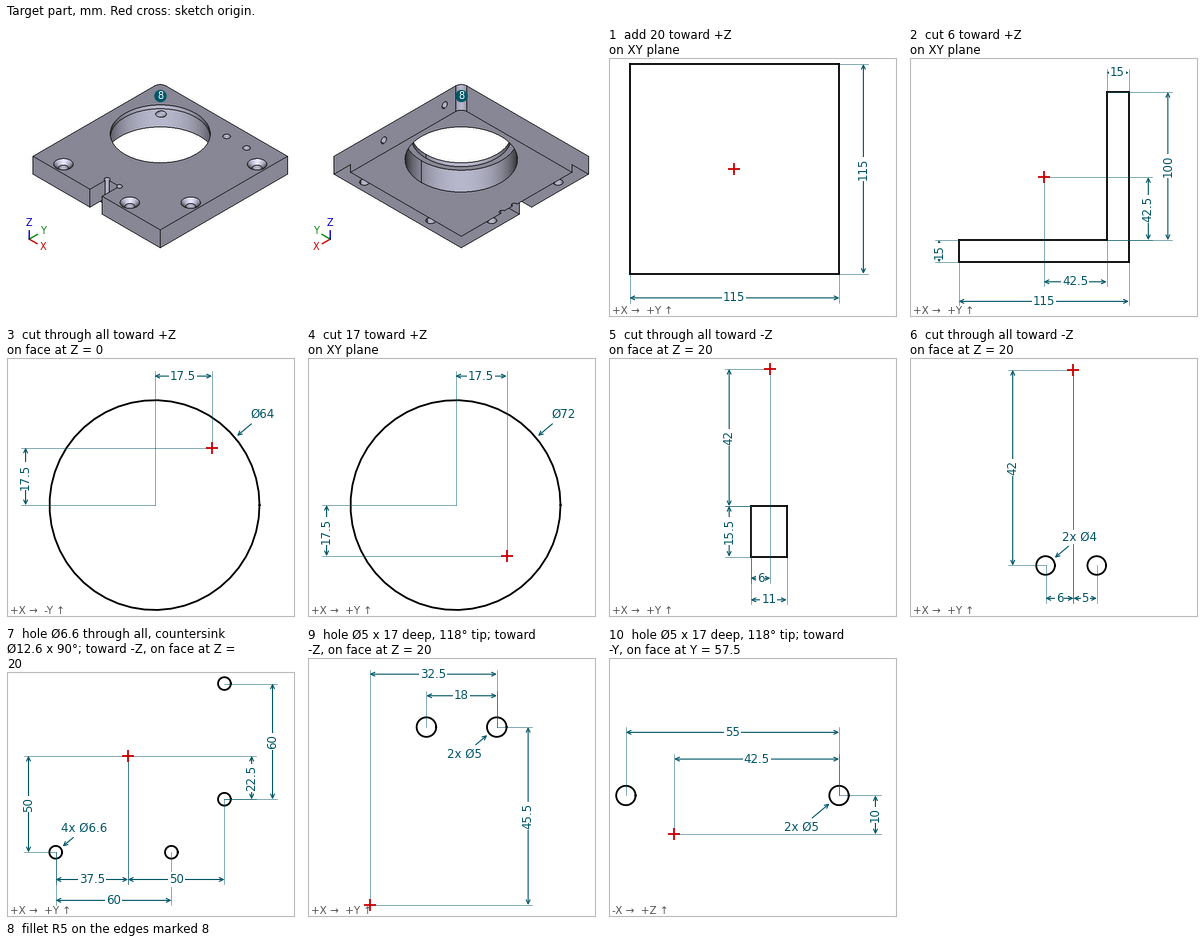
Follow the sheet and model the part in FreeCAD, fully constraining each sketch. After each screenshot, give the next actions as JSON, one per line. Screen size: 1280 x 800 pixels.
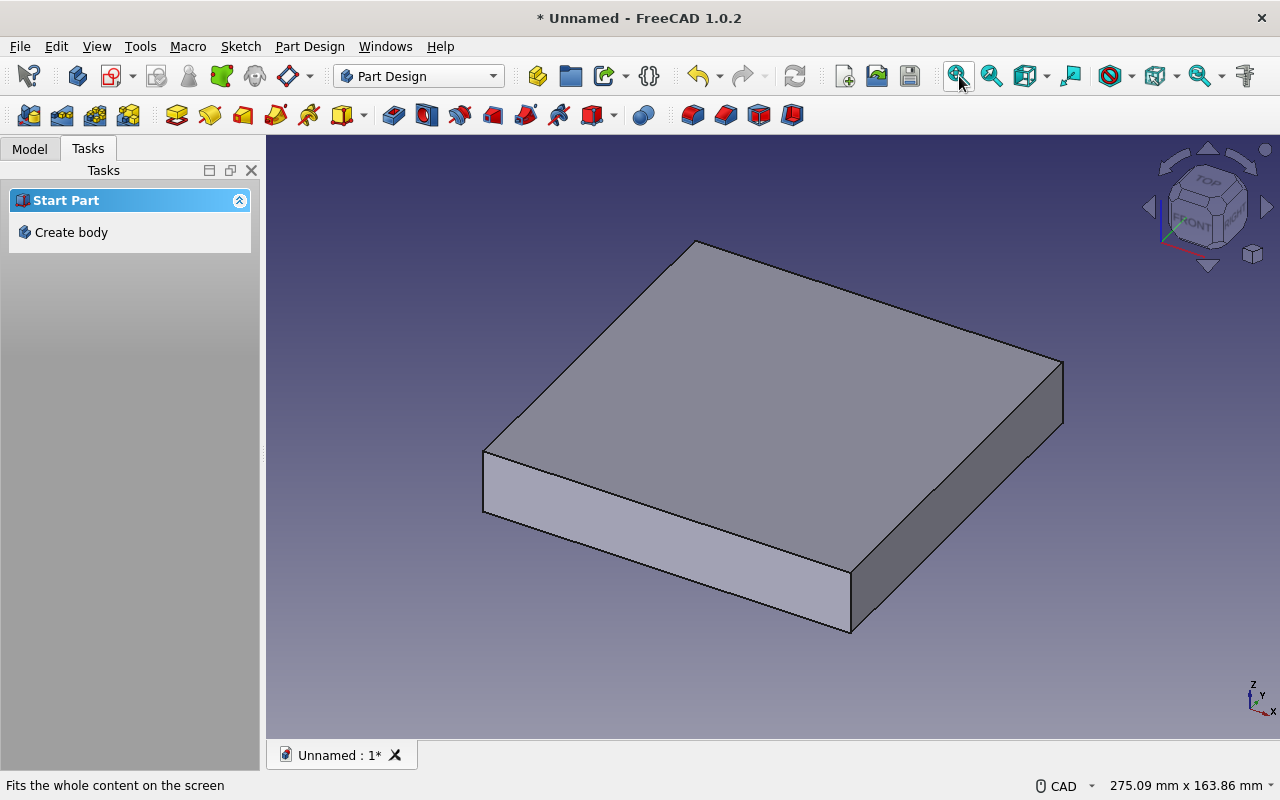
{"action": "left_click", "coordinate": [110, 76]}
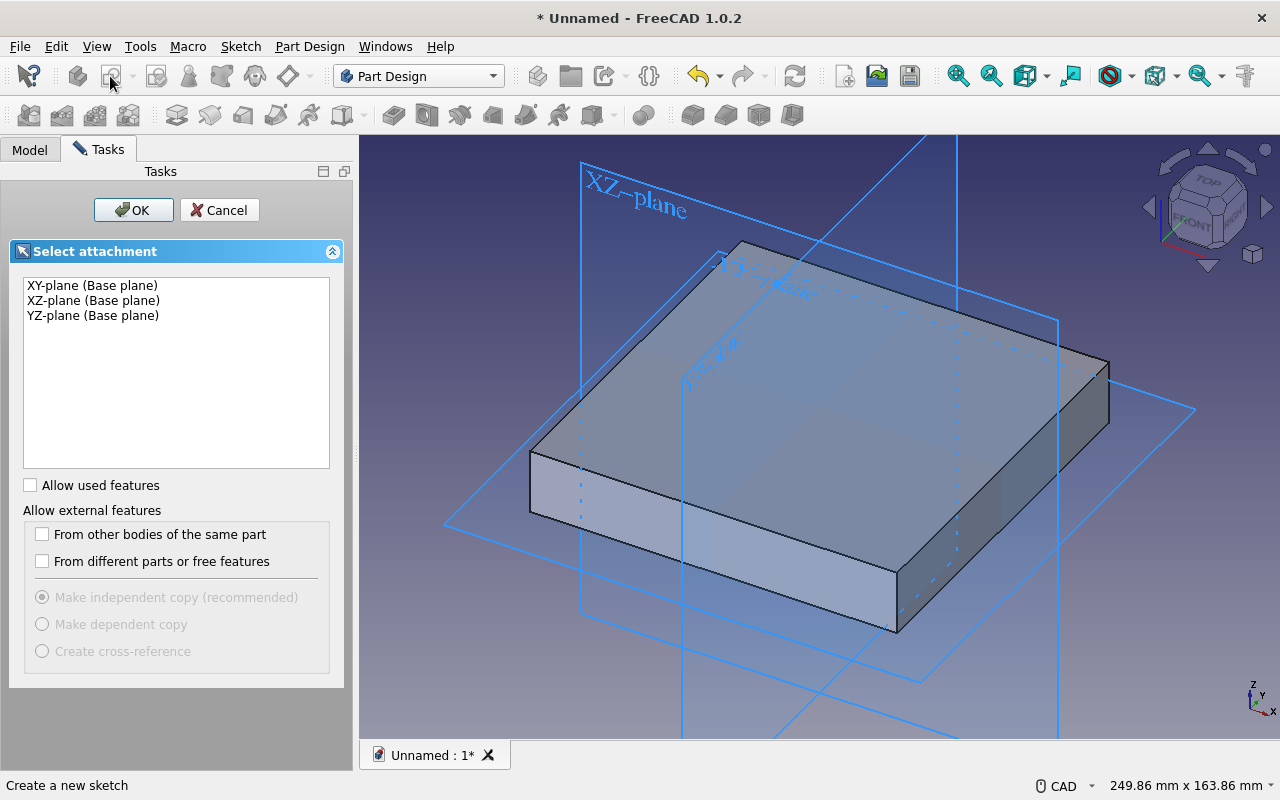
{"action": "left_click", "coordinate": [84, 286]}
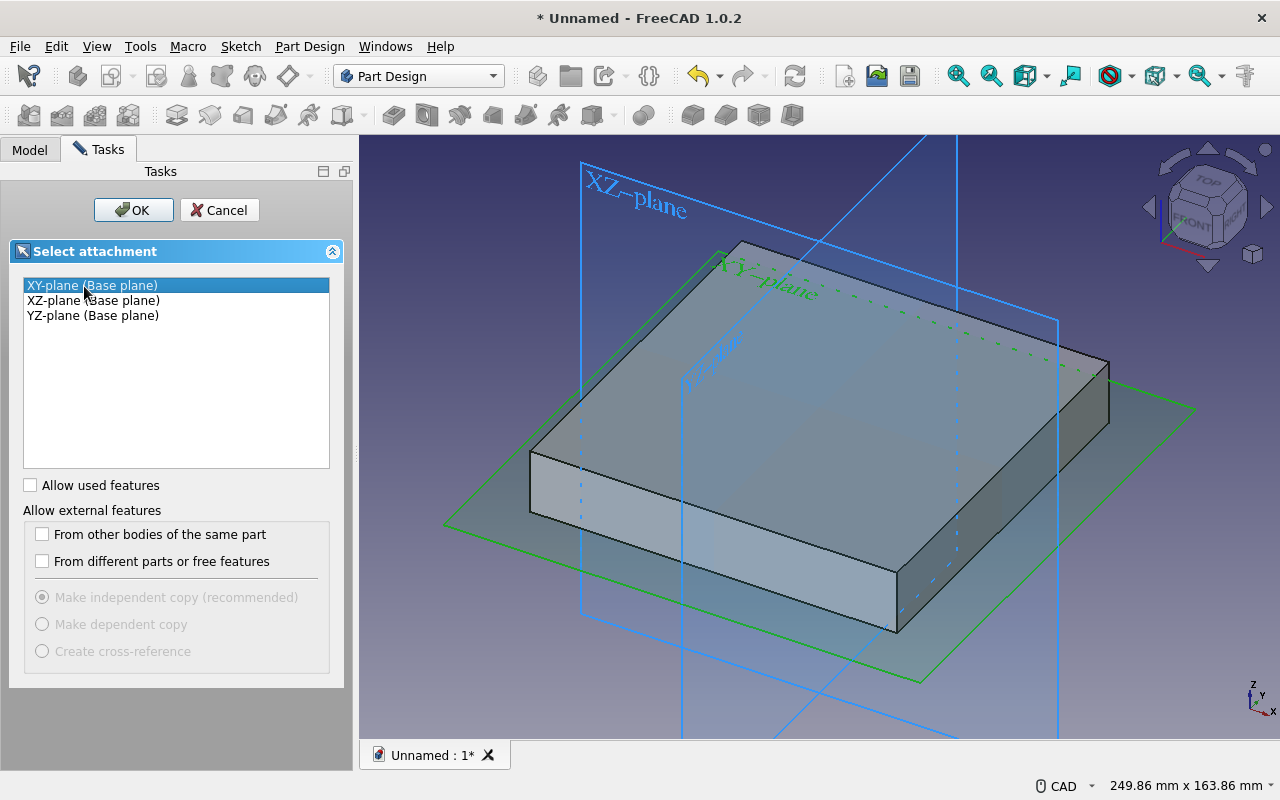
{"action": "left_click", "coordinate": [134, 210]}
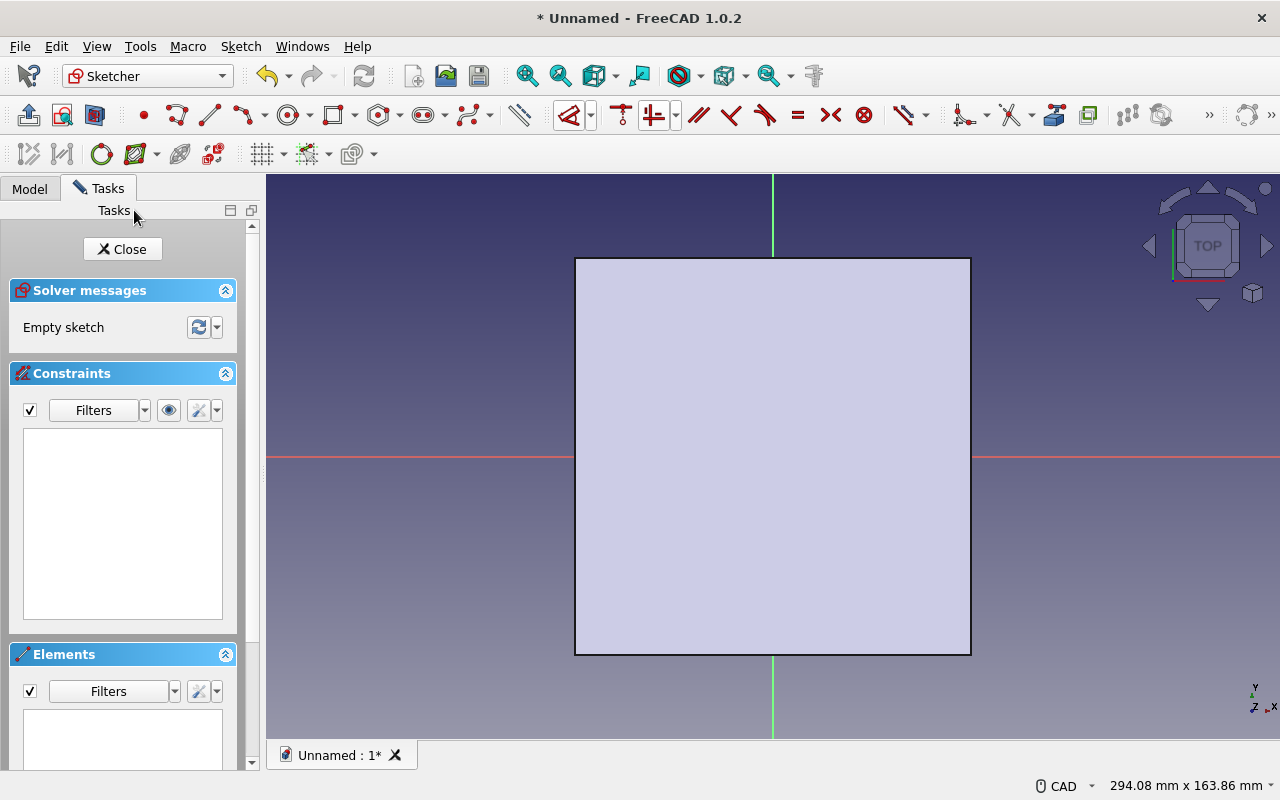
{"action": "key", "text": "q s"}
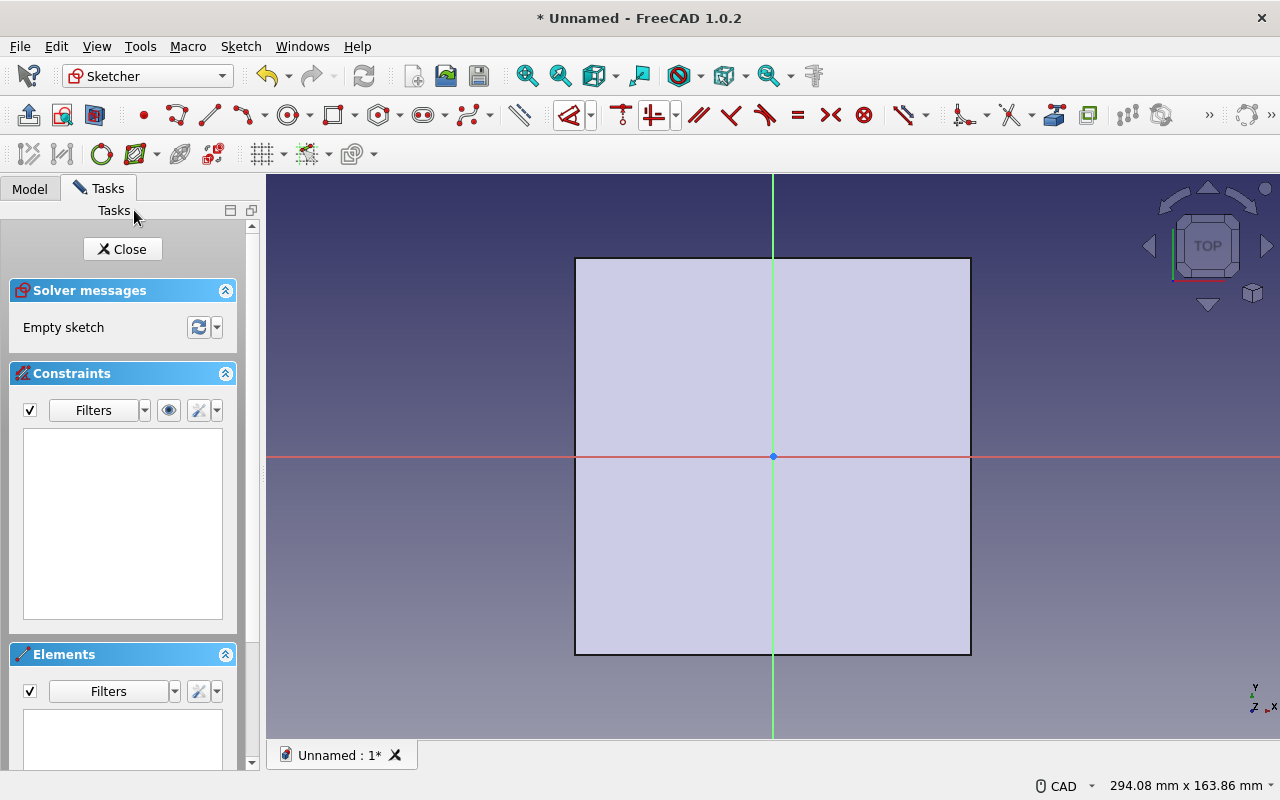
{"action": "key", "text": "g m"}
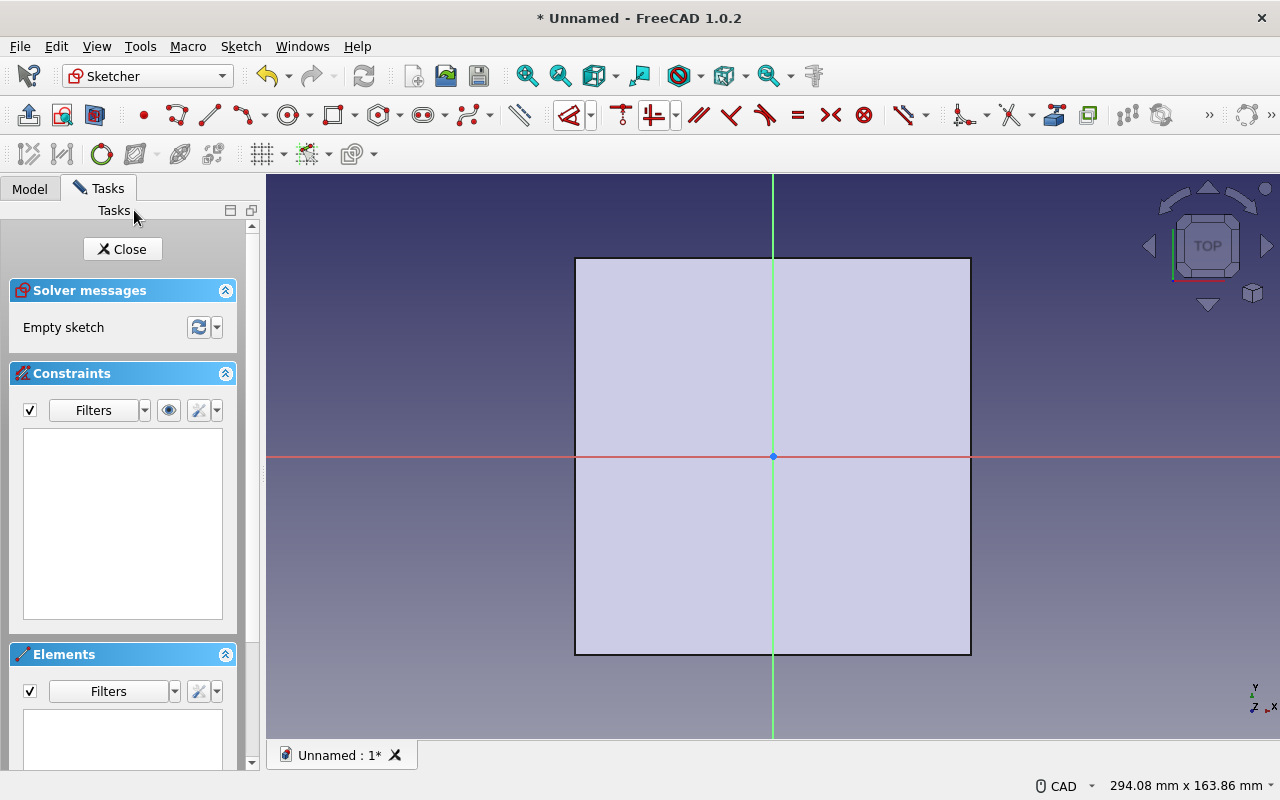
{"action": "left_click", "coordinate": [920, 603]}
{"action": "left_click", "coordinate": [920, 258]}
{"action": "left_click", "coordinate": [971, 258]}
{"action": "left_click", "coordinate": [971, 655]}
{"action": "left_click", "coordinate": [575, 655]}
{"action": "left_click", "coordinate": [575, 603]}
{"action": "left_click", "coordinate": [920, 604]}
{"action": "key", "text": "Escape"}
{"action": "key", "text": "Escape"}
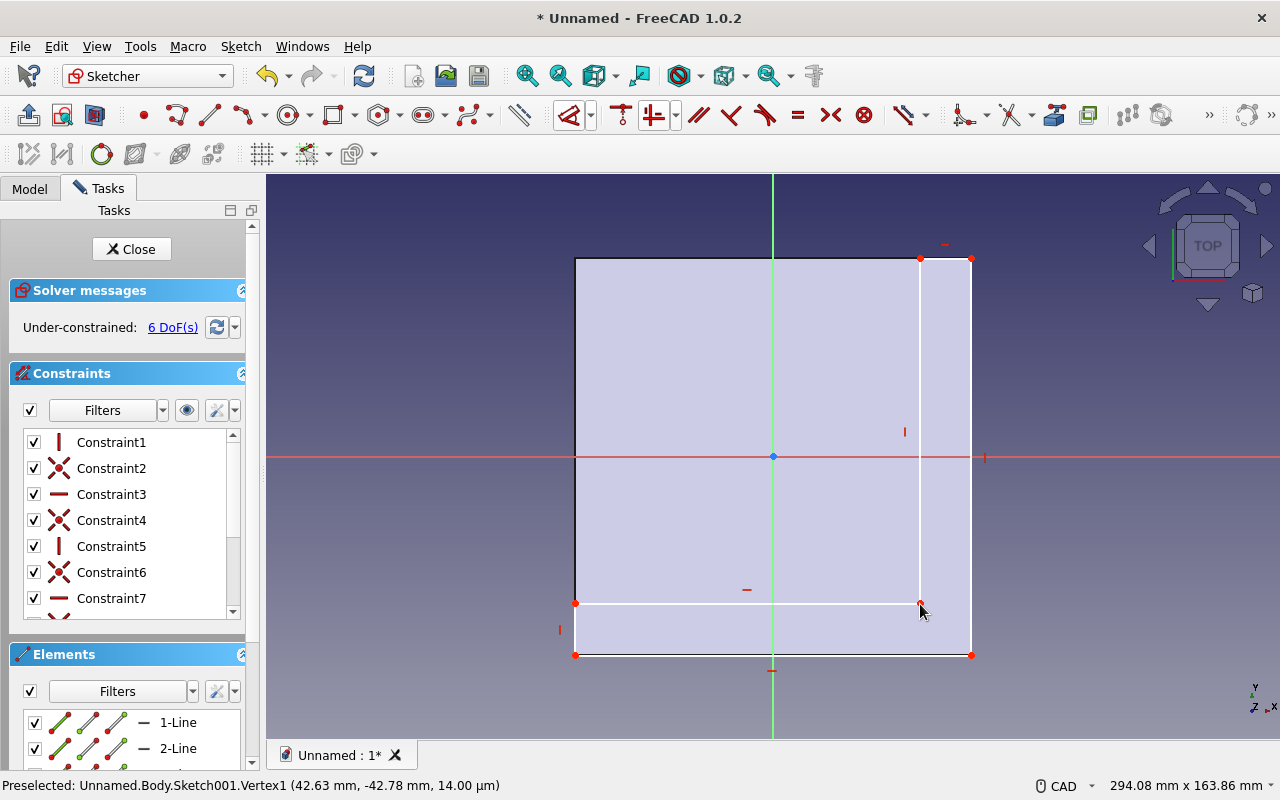
{"action": "left_click", "coordinate": [935, 259]}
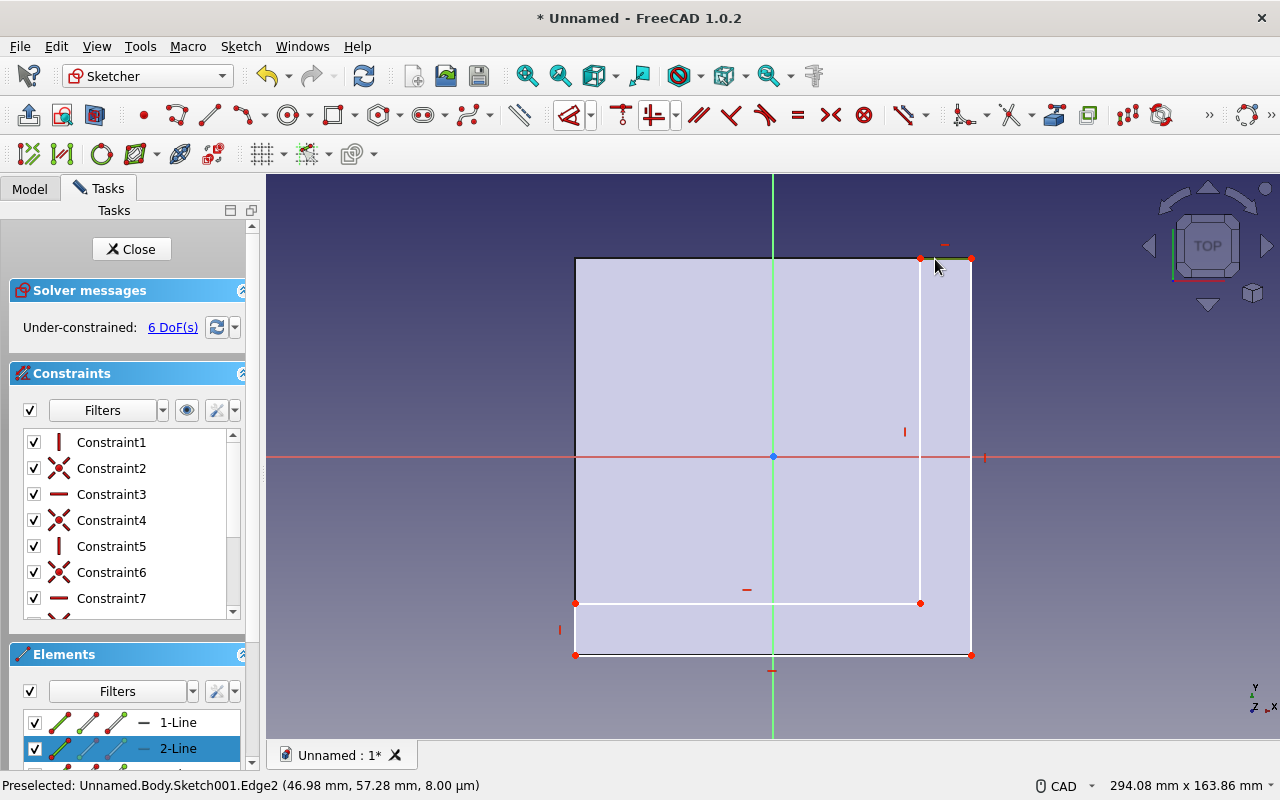
{"action": "left_click", "coordinate": [590, 116]}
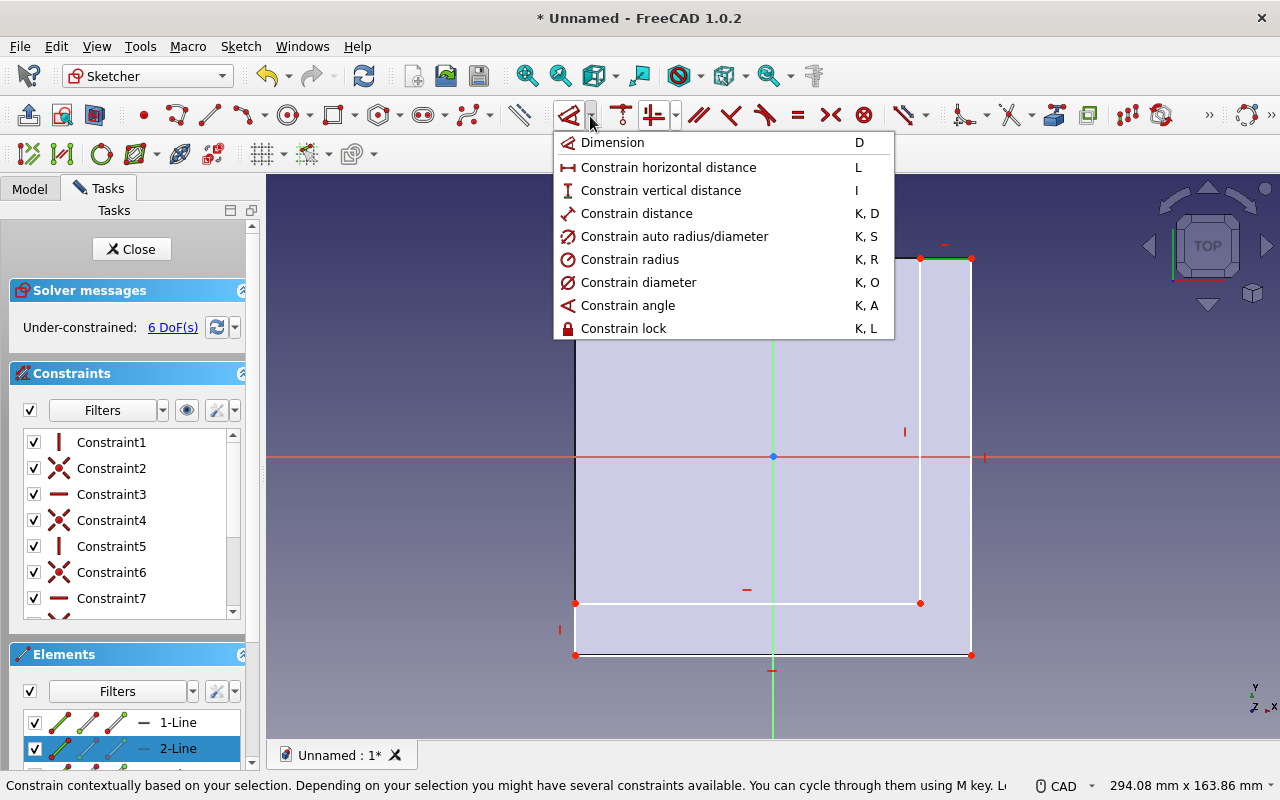
{"action": "left_click", "coordinate": [724, 168]}